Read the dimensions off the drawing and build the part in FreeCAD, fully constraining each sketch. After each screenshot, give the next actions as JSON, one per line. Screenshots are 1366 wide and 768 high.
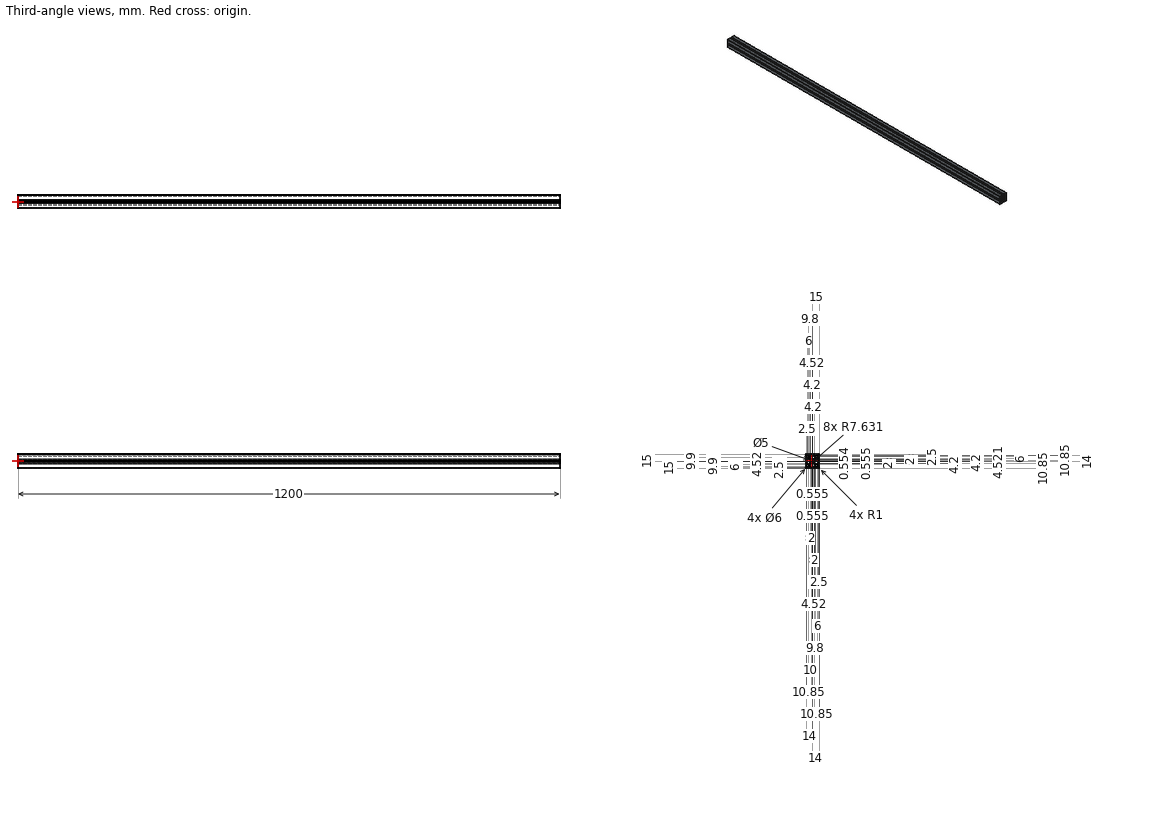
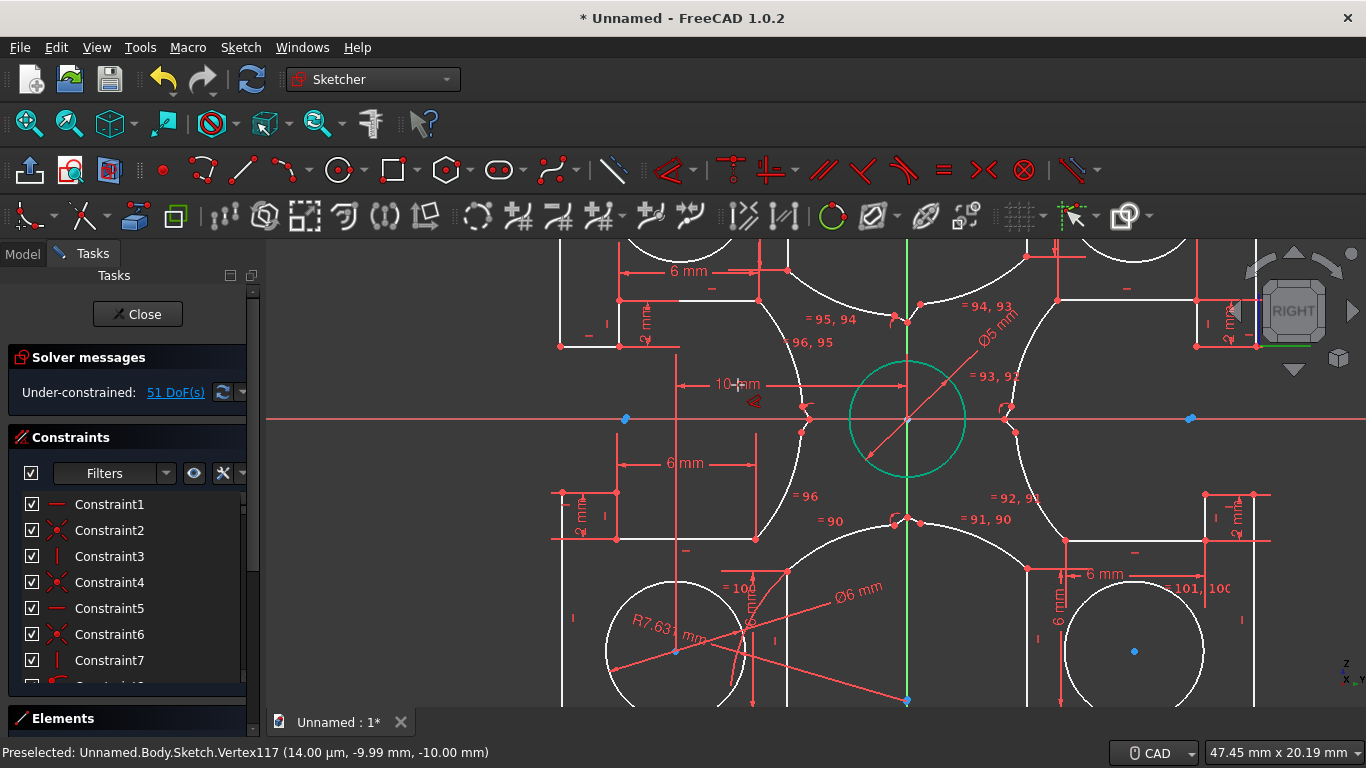
{"action": "scroll", "coordinate": [617, 517], "scroll_direction": "down", "scroll_amount": 4}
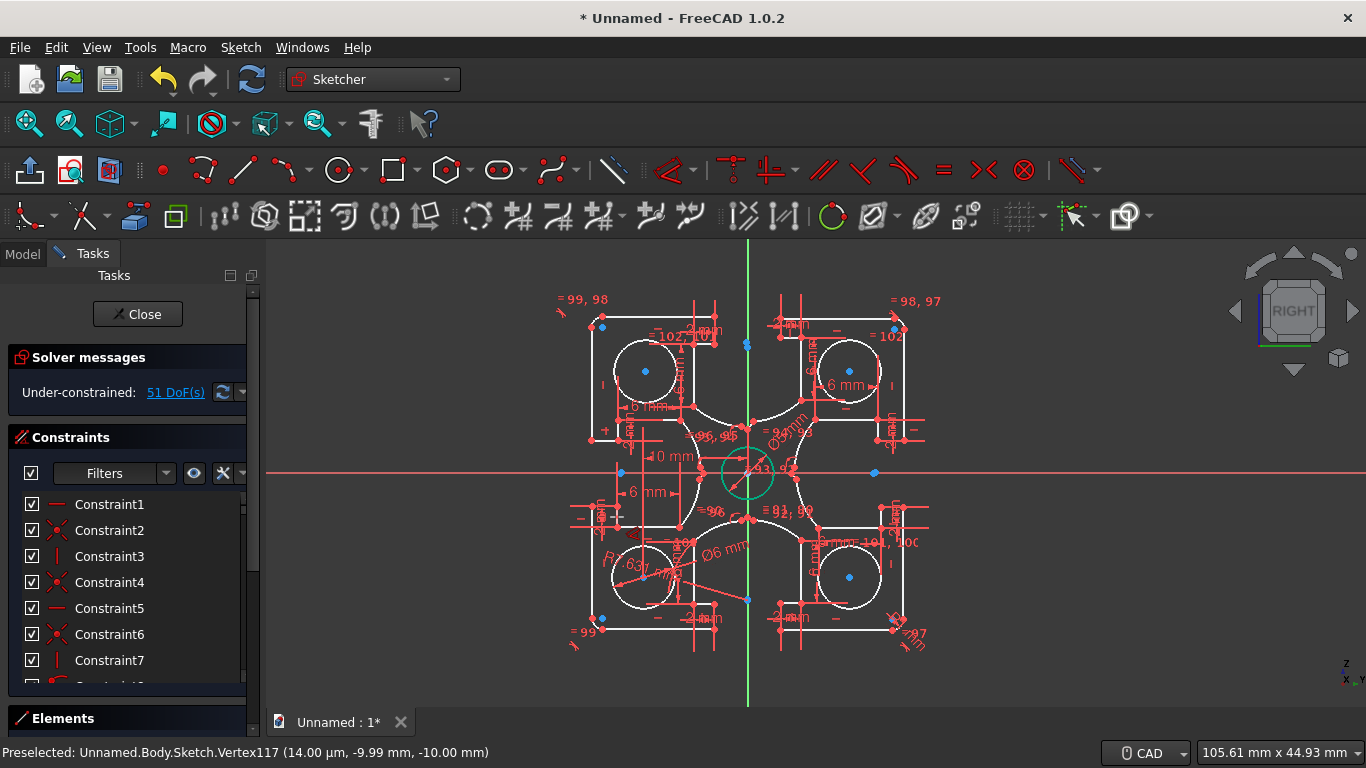
{"action": "scroll", "coordinate": [714, 622], "scroll_direction": "up", "scroll_amount": 4}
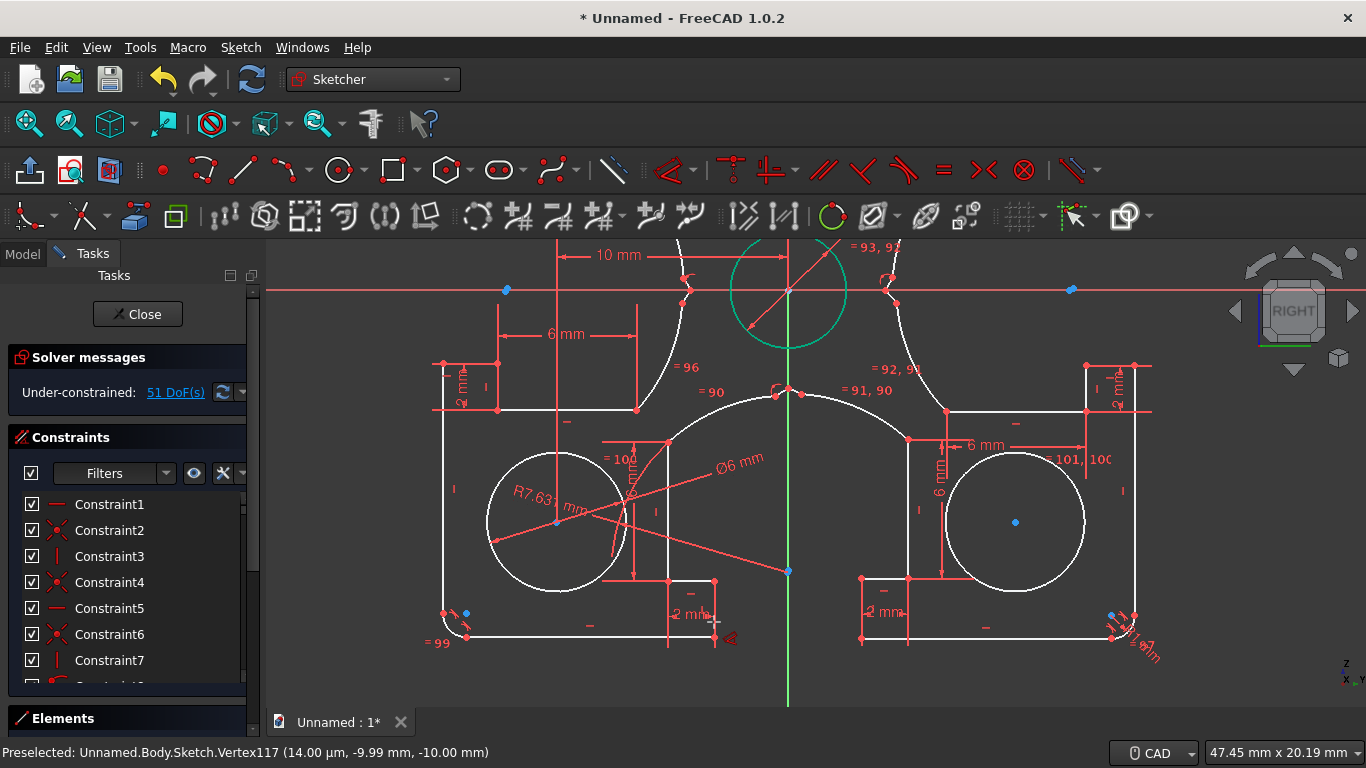
{"action": "left_click", "coordinate": [715, 620]}
{"action": "left_click", "coordinate": [681, 596]}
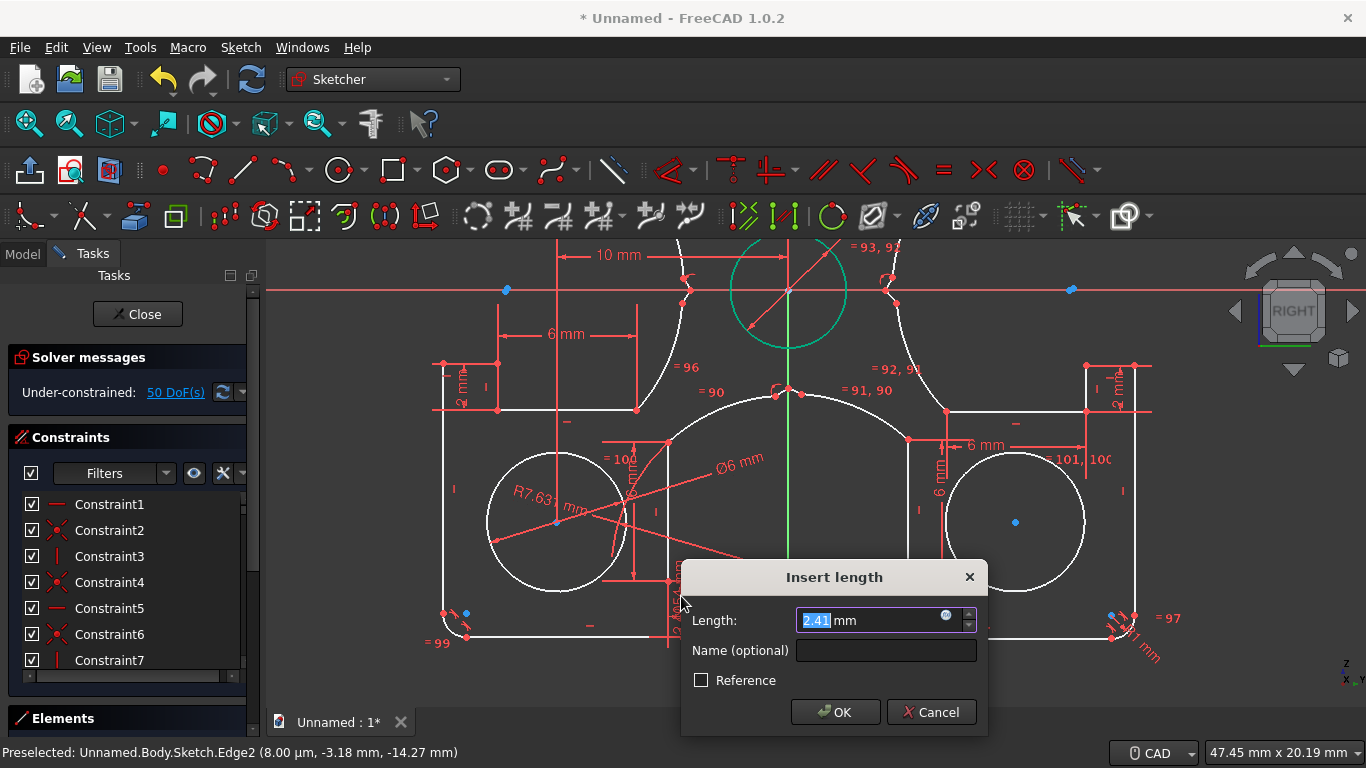
{"action": "type", "text": "2.5"}
{"action": "key", "text": "Return"}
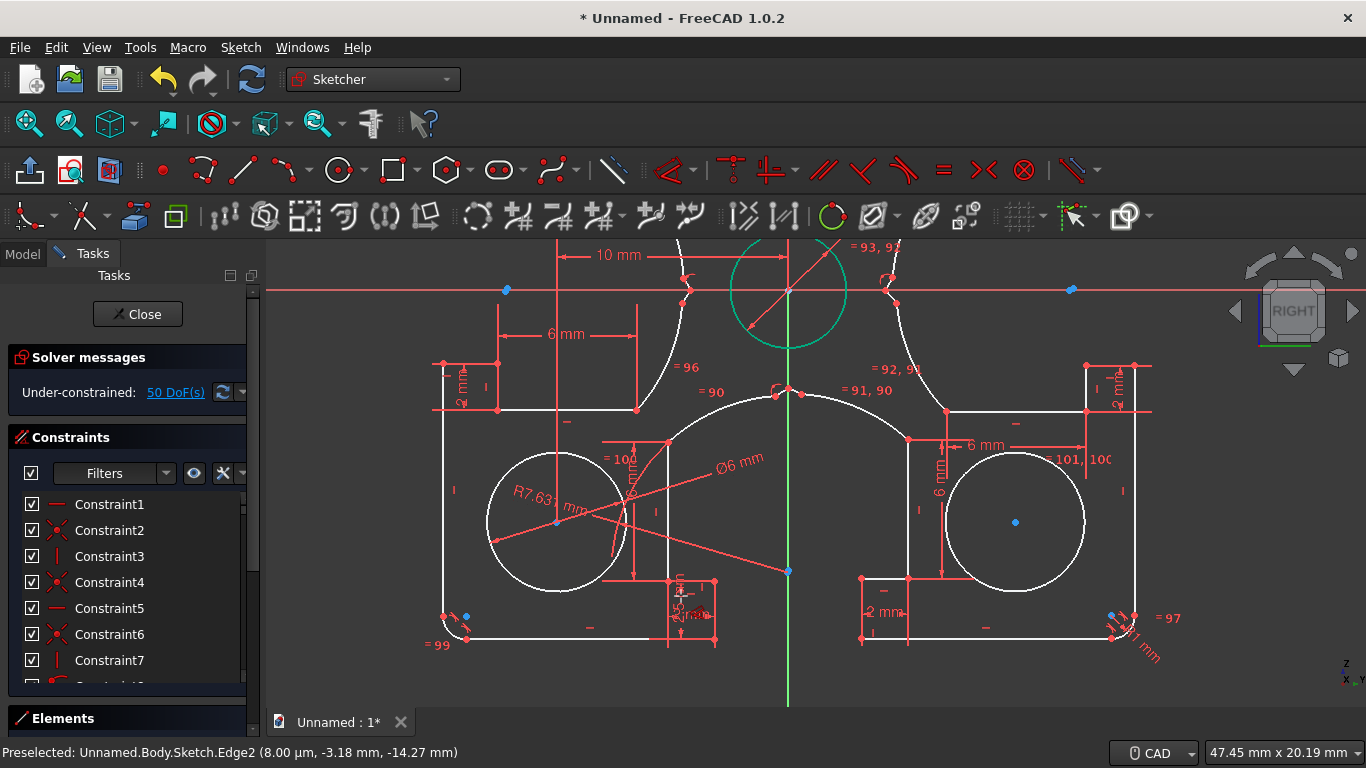
{"action": "left_click", "coordinate": [862, 597]}
{"action": "left_click", "coordinate": [828, 588]}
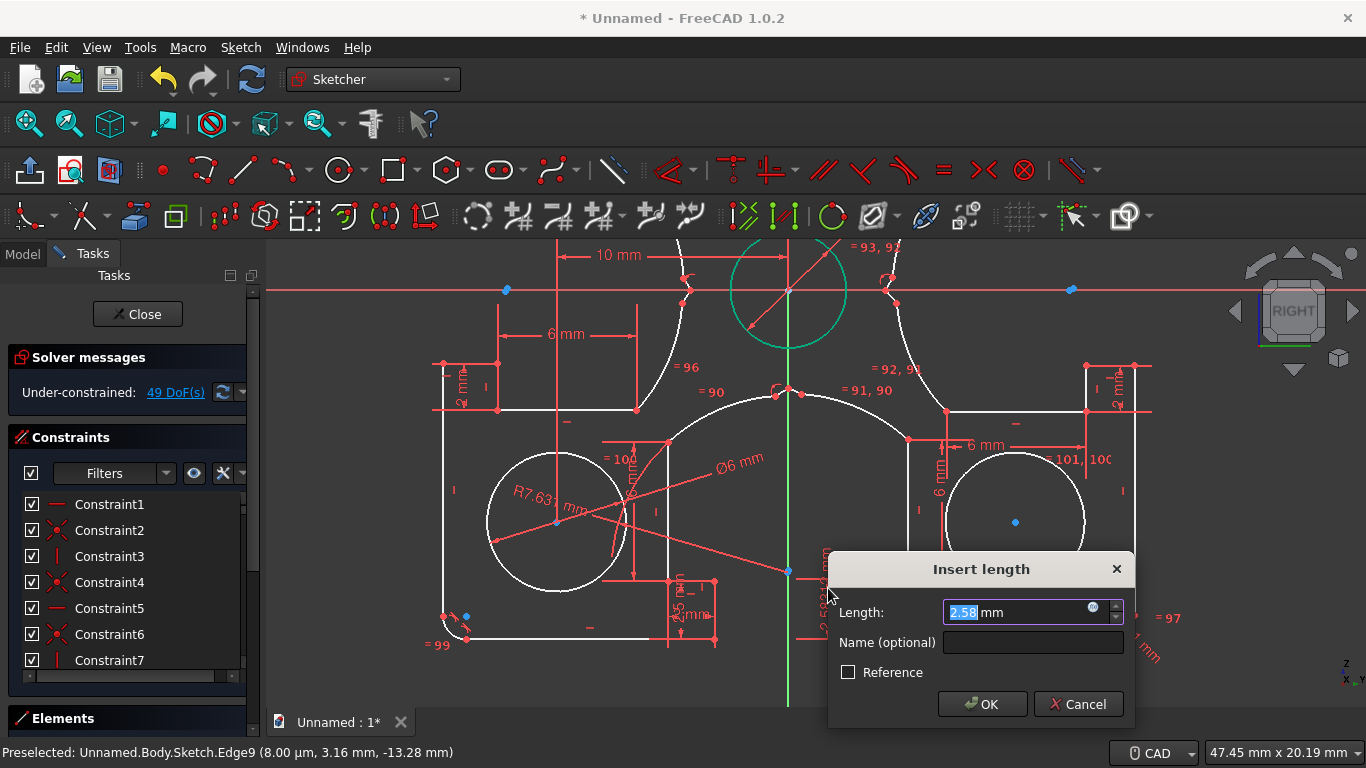
{"action": "type", "text": "2.5"}
{"action": "key", "text": "Return"}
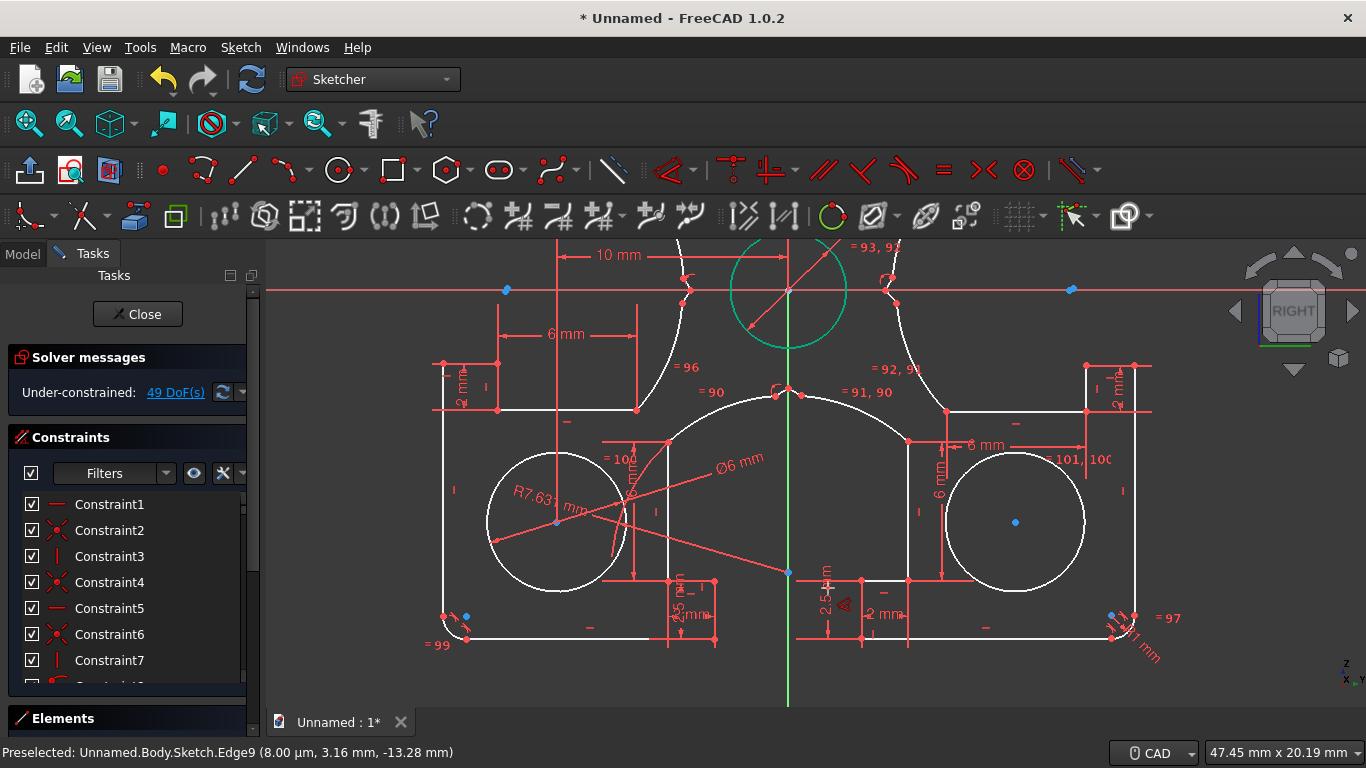
{"action": "left_click", "coordinate": [1120, 366]}
{"action": "left_click", "coordinate": [1110, 332]}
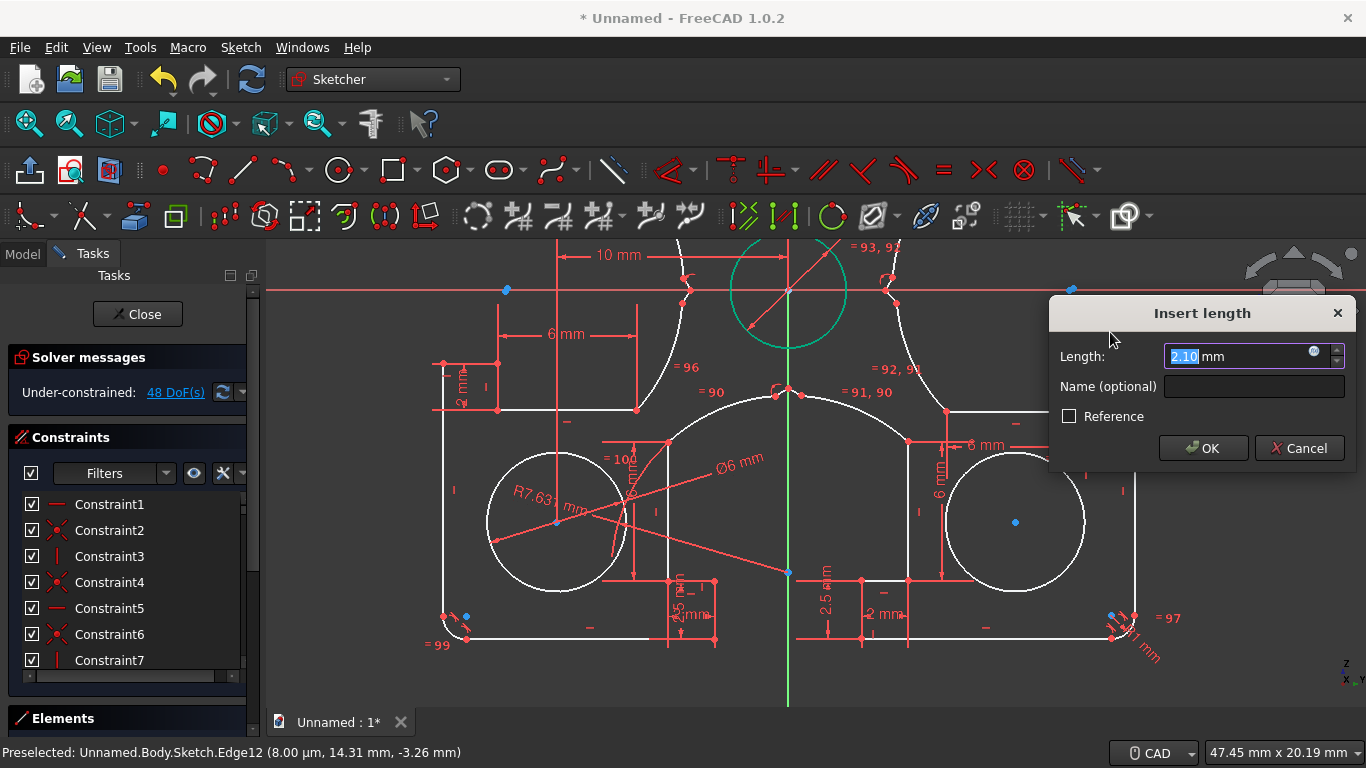
{"action": "type", "text": "2.5"}
{"action": "key", "text": "Return"}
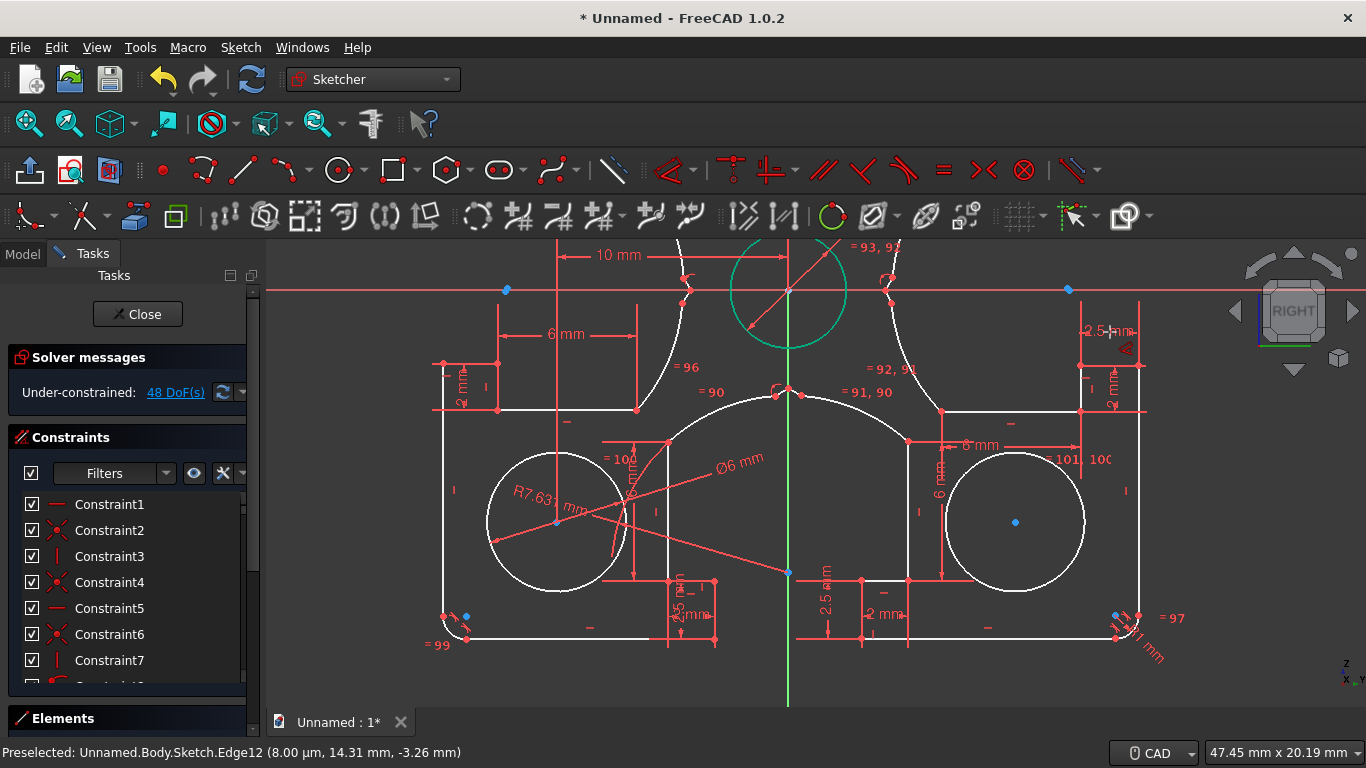
{"action": "scroll", "coordinate": [714, 622], "scroll_direction": "down", "scroll_amount": 4}